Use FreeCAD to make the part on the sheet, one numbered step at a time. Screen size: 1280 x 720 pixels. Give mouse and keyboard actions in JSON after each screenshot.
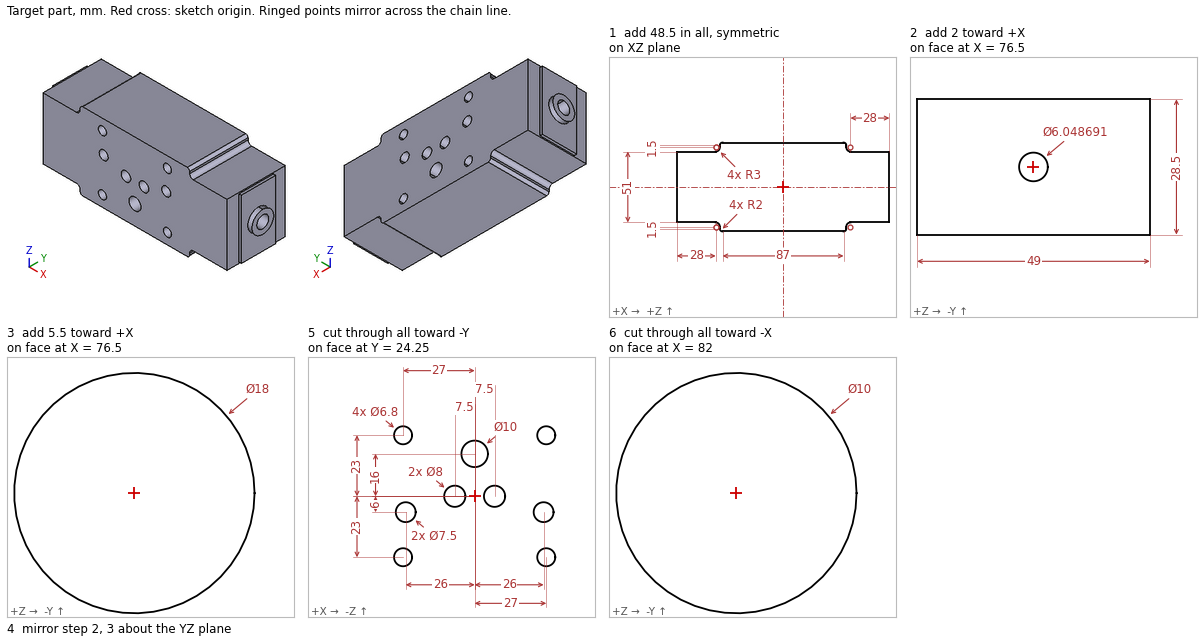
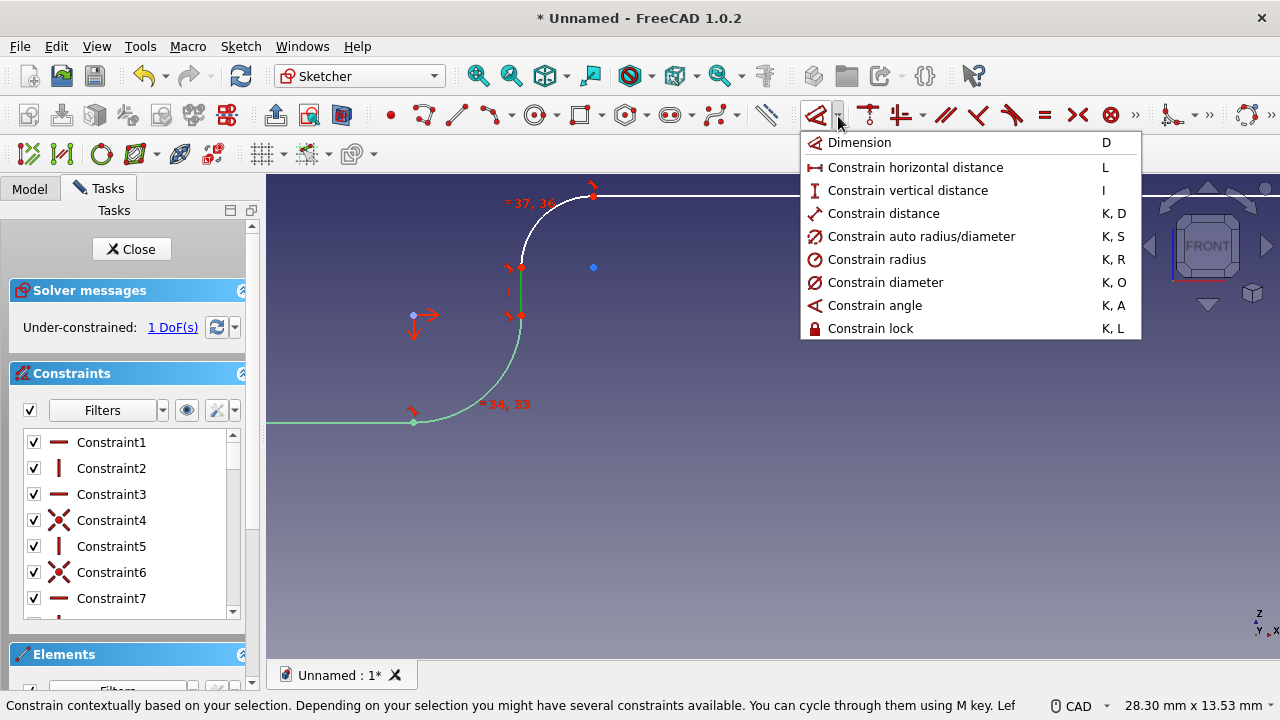
{"action": "left_click", "coordinate": [971, 190]}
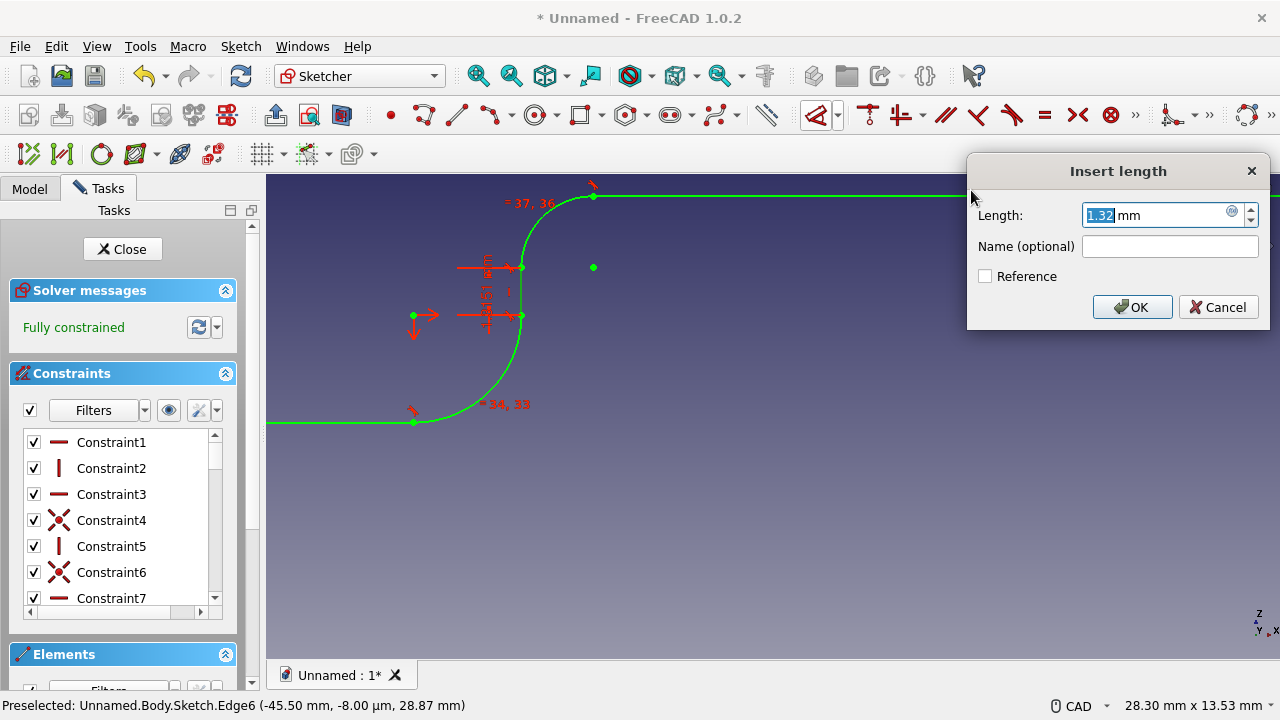
{"action": "type", "text": "1.5"}
{"action": "key", "text": "Return"}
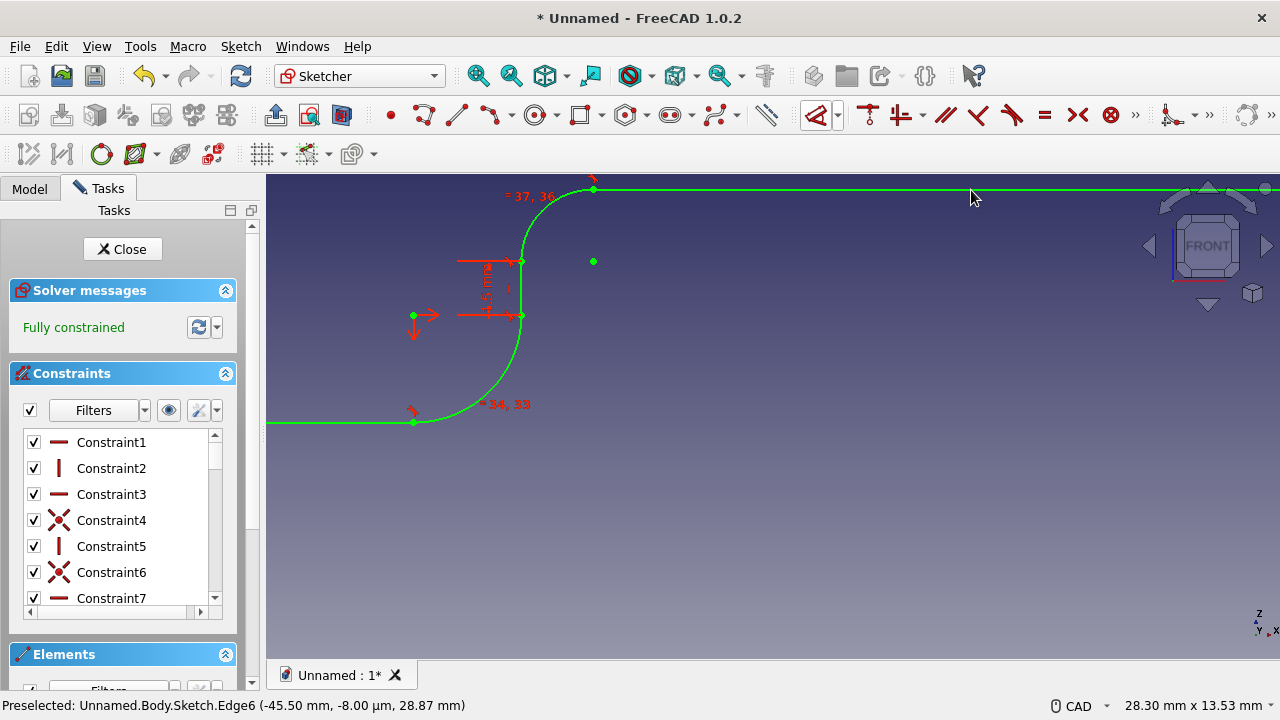
{"action": "left_click", "coordinate": [123, 249]}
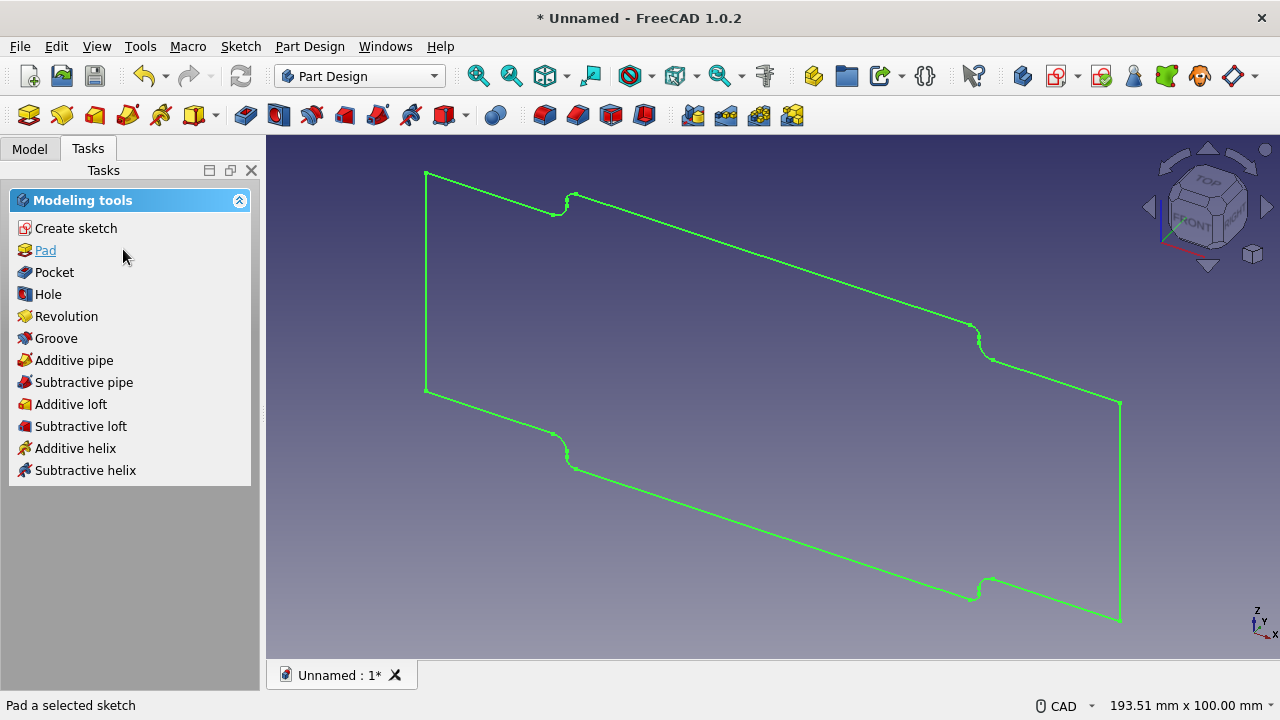
{"action": "left_click", "coordinate": [29, 116]}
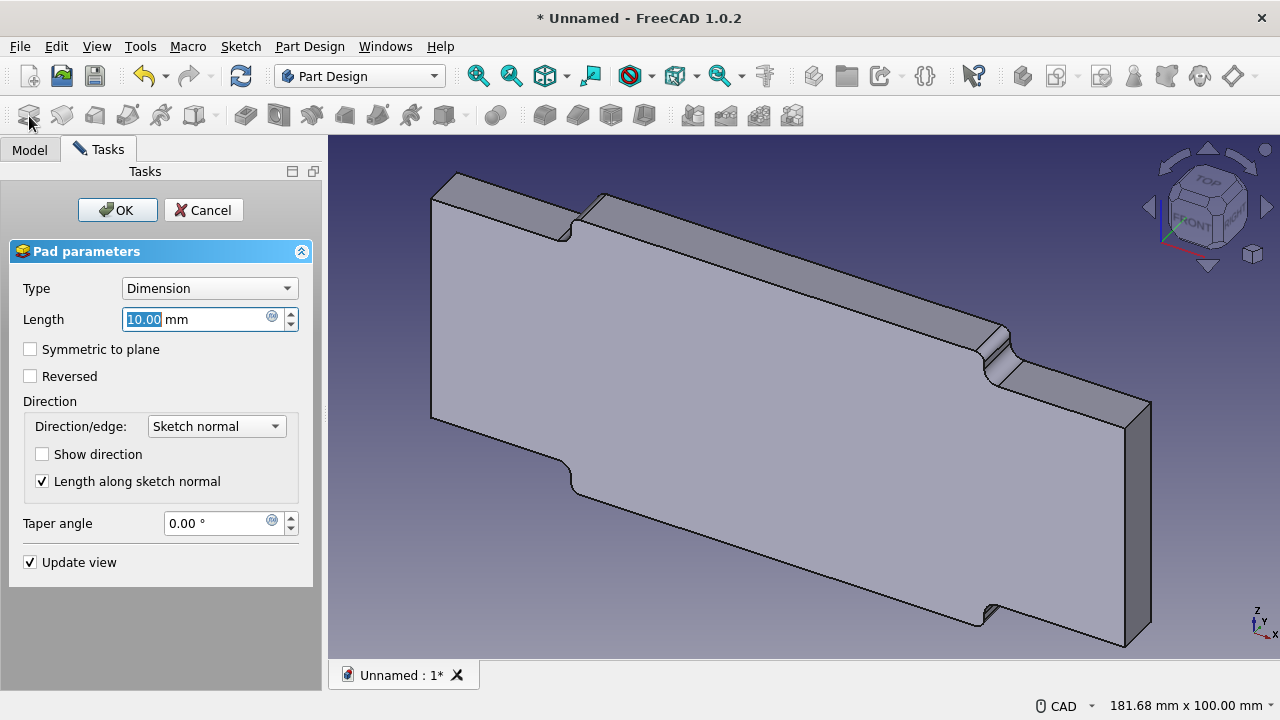
{"action": "type", "text": "48.5"}
{"action": "key", "text": "Tab"}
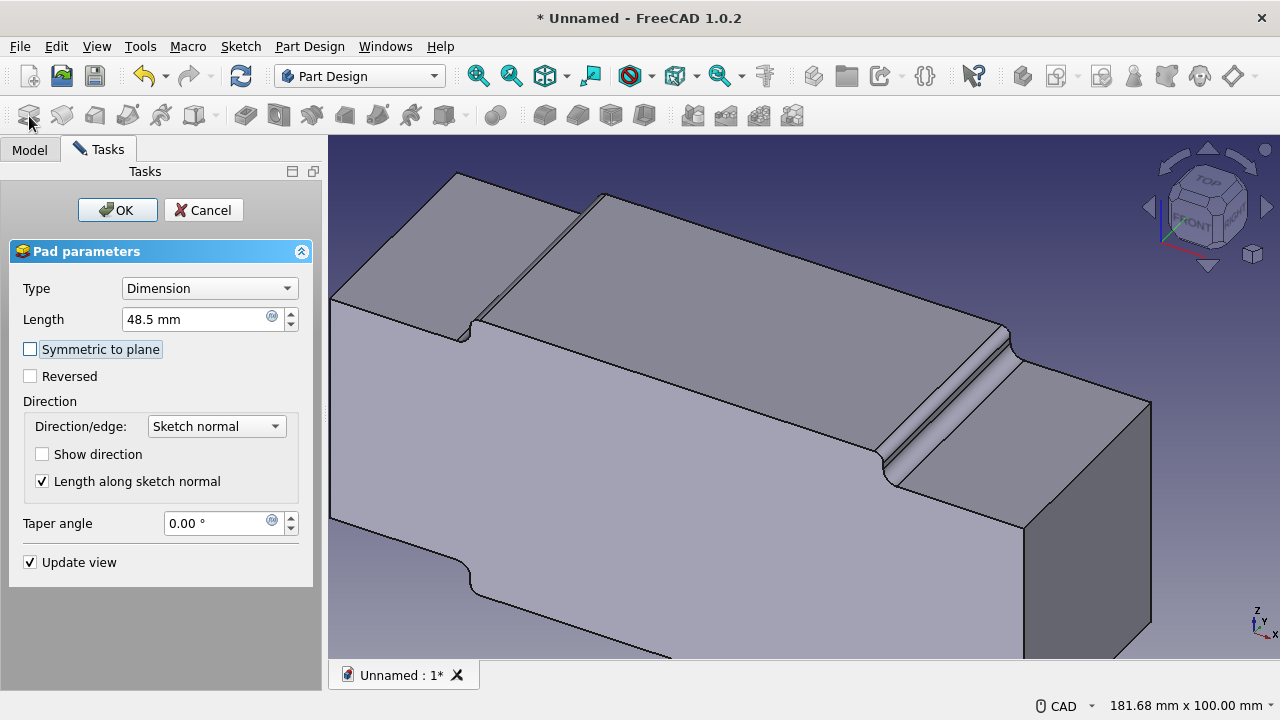
{"action": "left_click", "coordinate": [31, 349]}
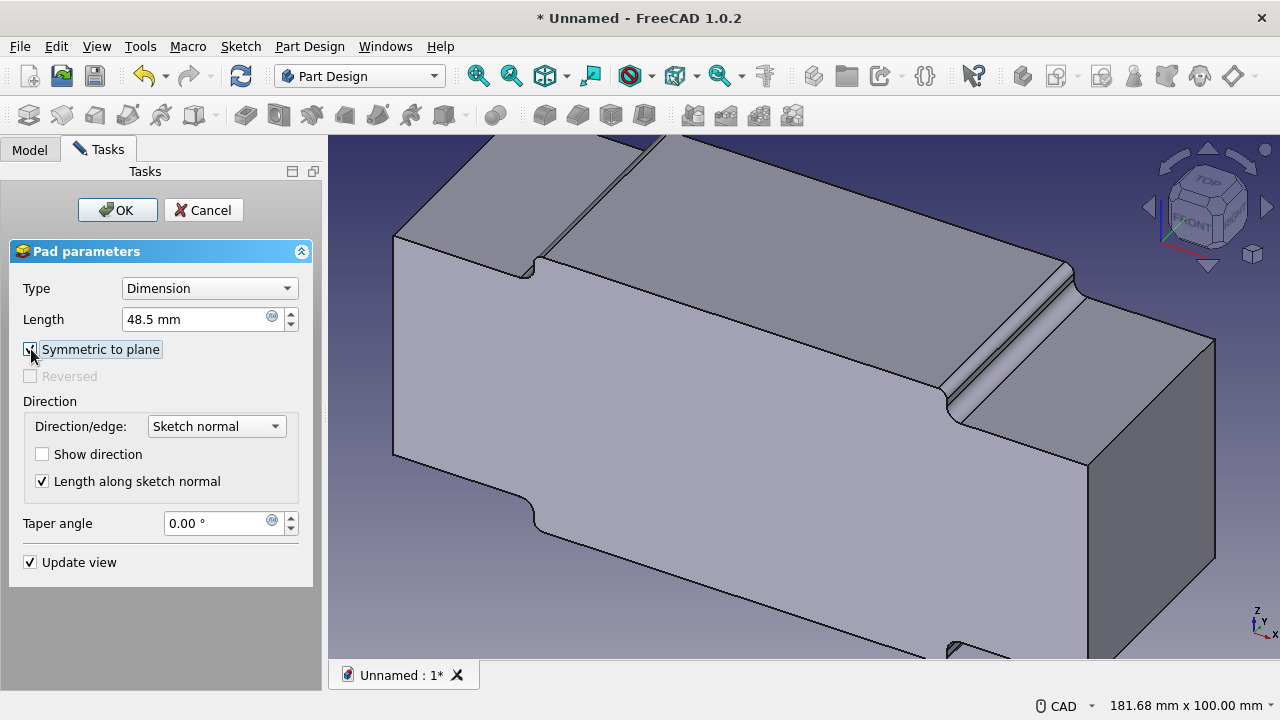
{"action": "left_click", "coordinate": [118, 210]}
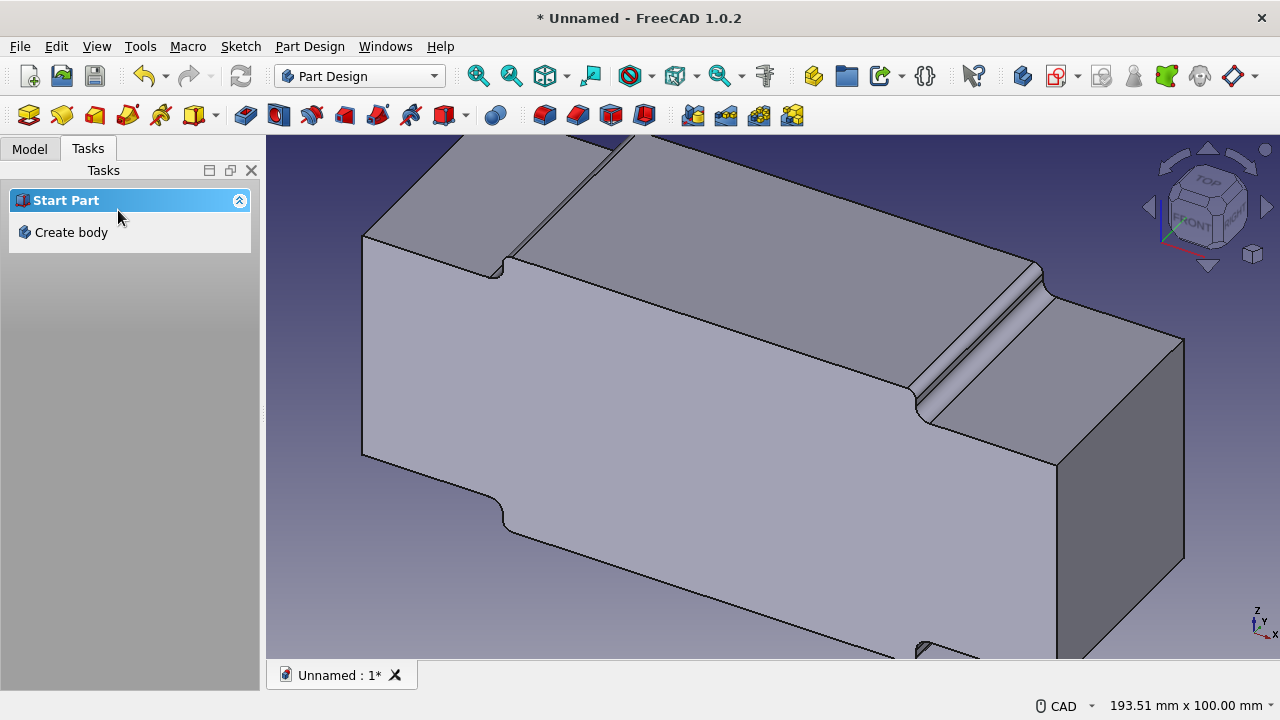
{"action": "left_click", "coordinate": [479, 76]}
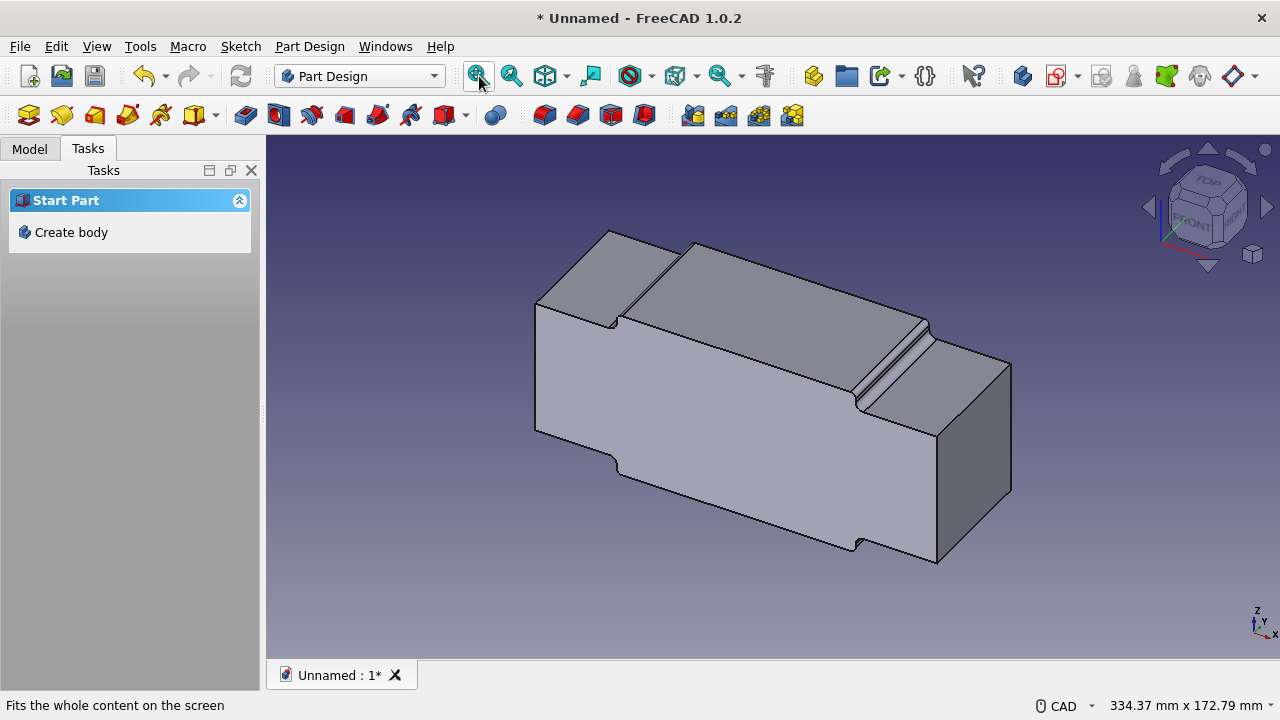
{"action": "left_click", "coordinate": [974, 463]}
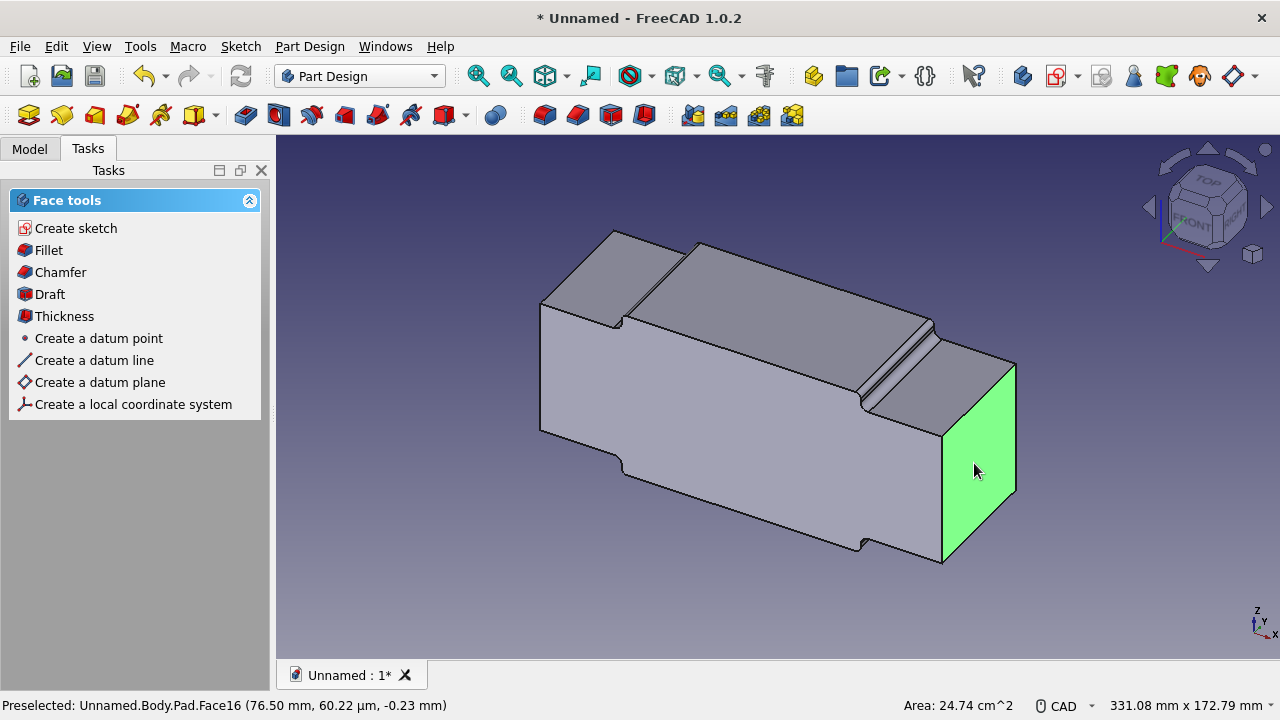
{"action": "left_click", "coordinate": [1056, 76]}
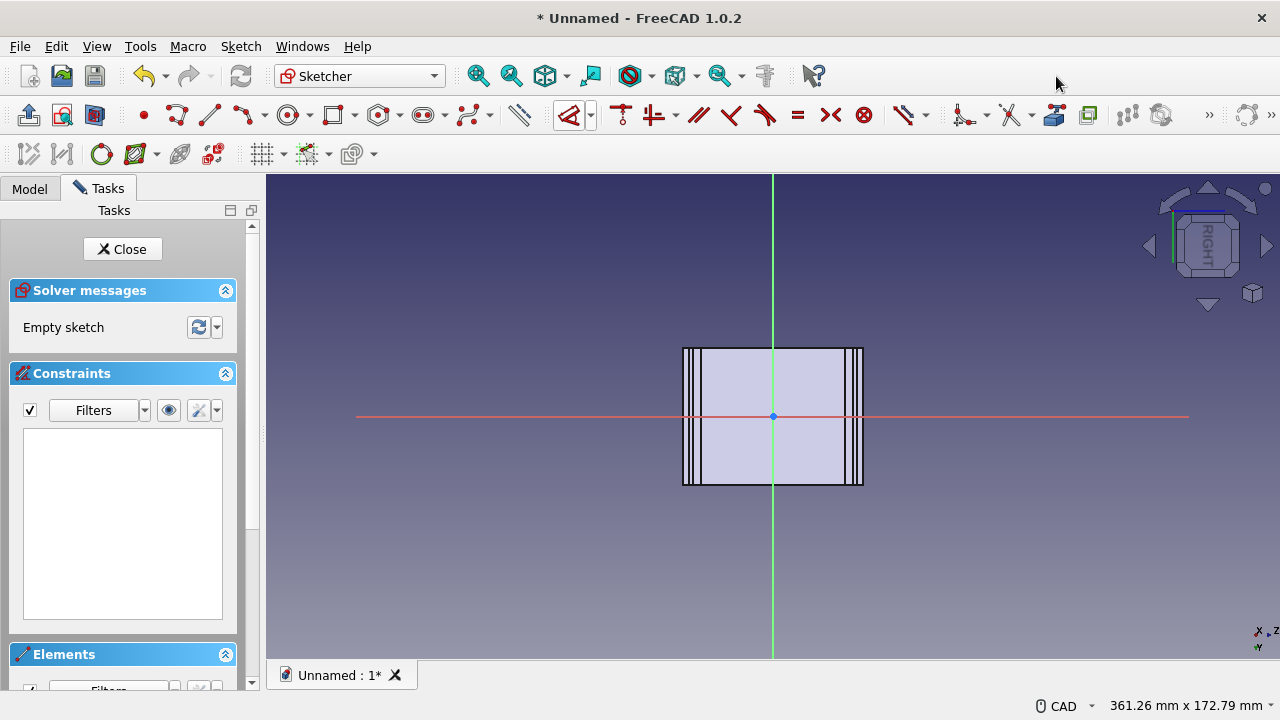
{"action": "scroll", "coordinate": [795, 416], "scroll_direction": "up", "scroll_amount": 7}